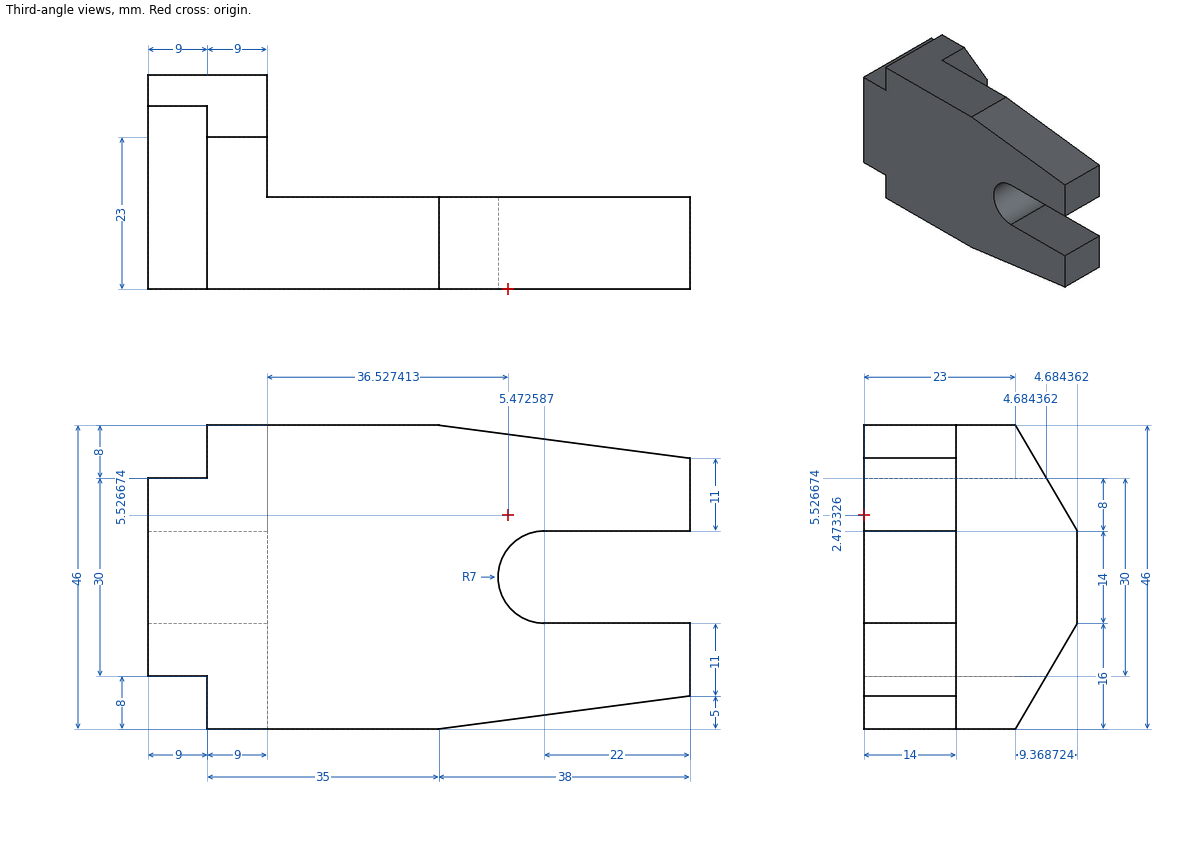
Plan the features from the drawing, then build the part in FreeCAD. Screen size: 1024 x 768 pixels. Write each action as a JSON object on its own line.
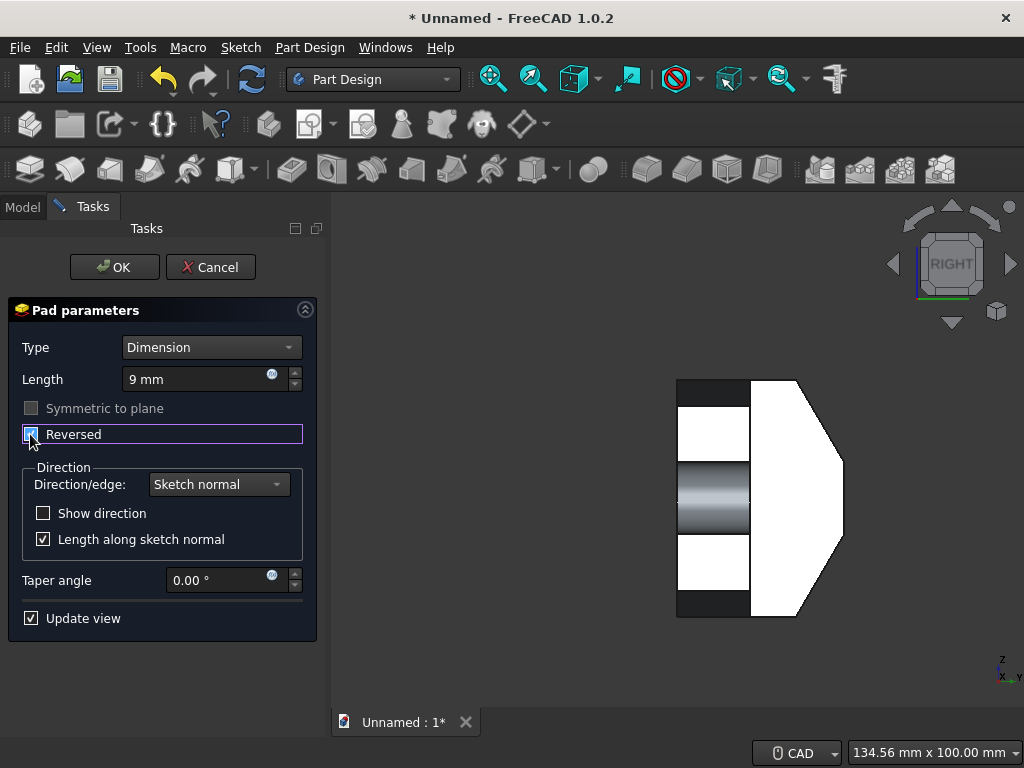
{"action": "left_click", "coordinate": [115, 267]}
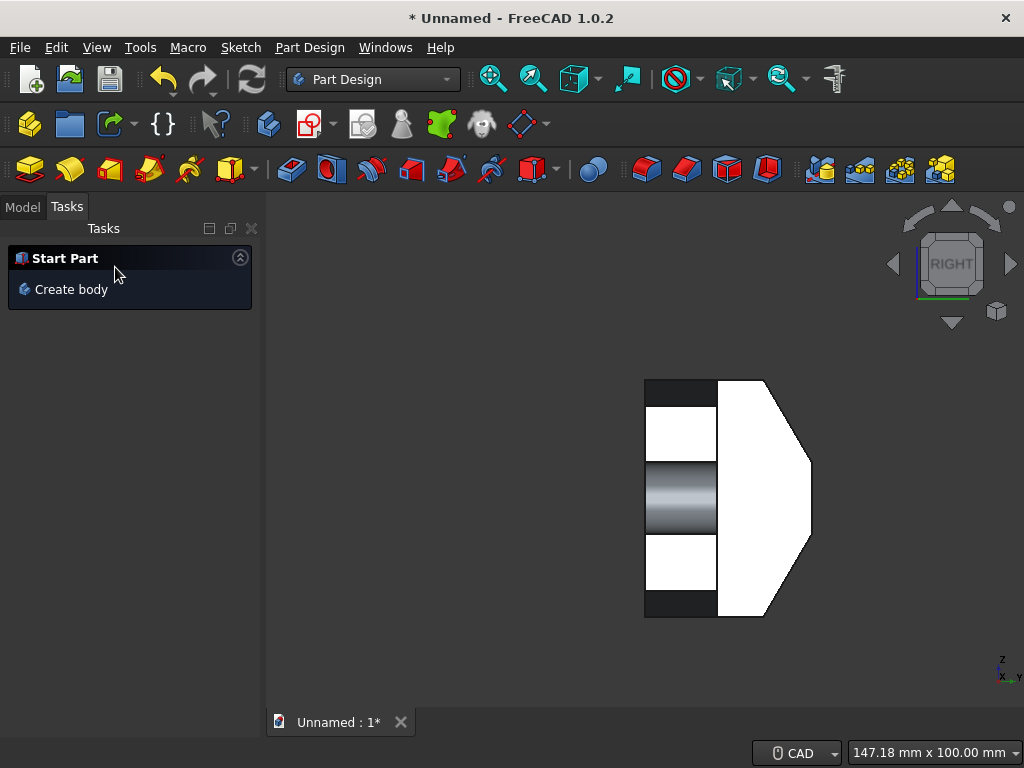
{"action": "key", "text": "6"}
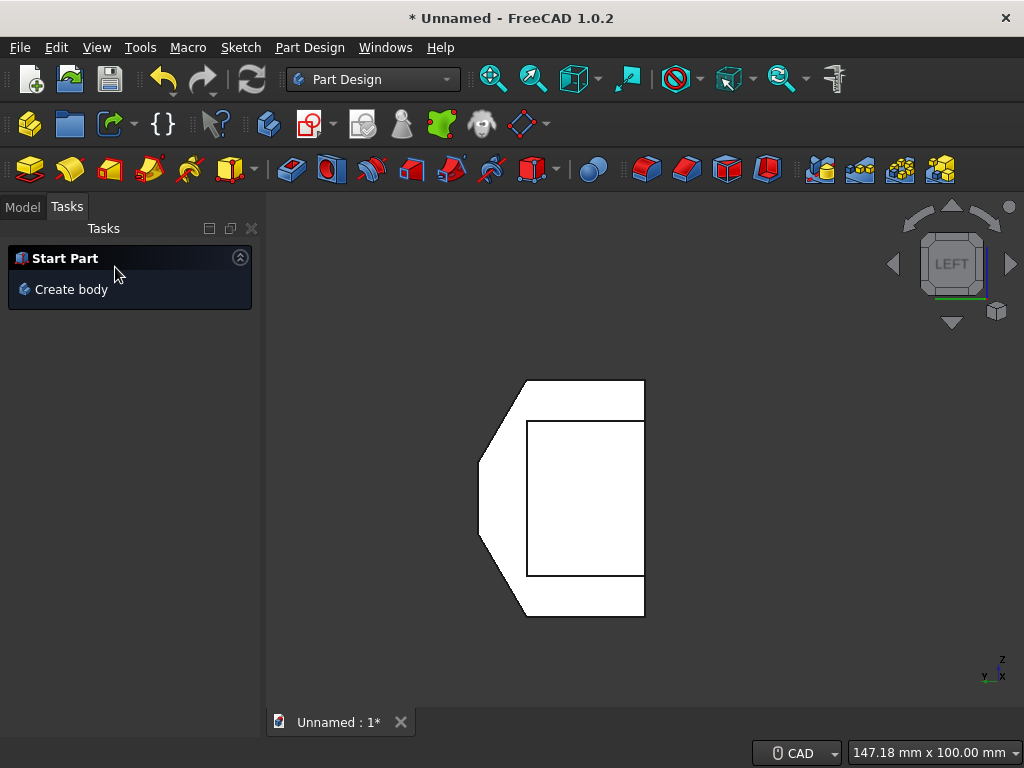
{"action": "left_click", "coordinate": [538, 599]}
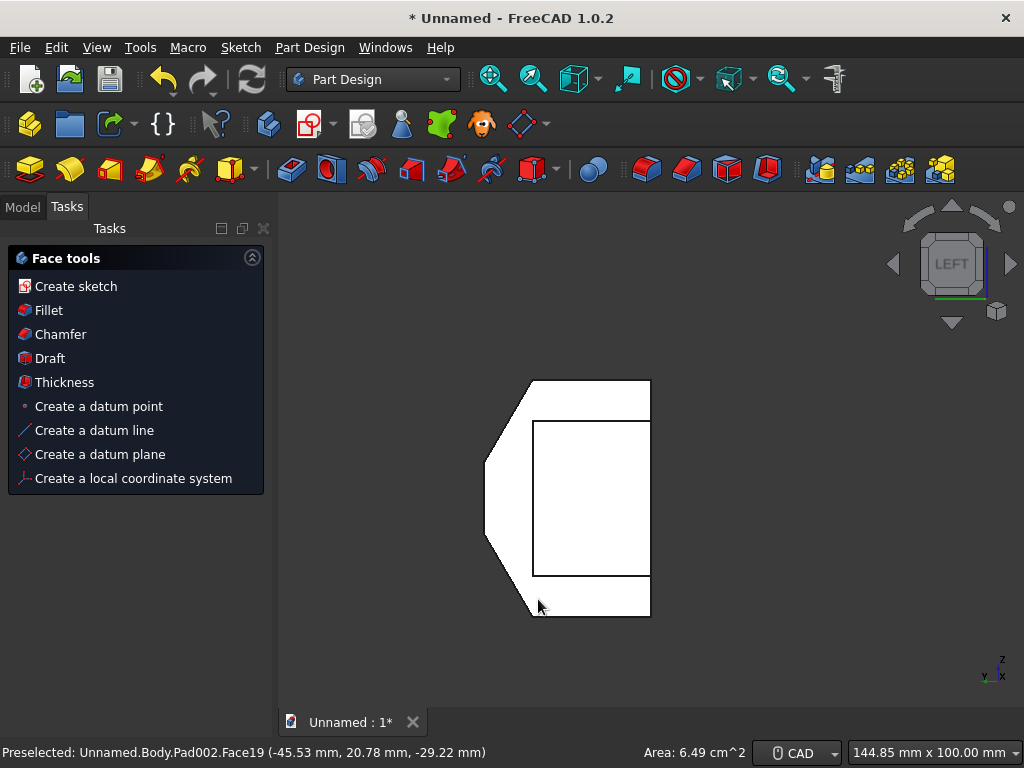
{"action": "left_click", "coordinate": [310, 124]}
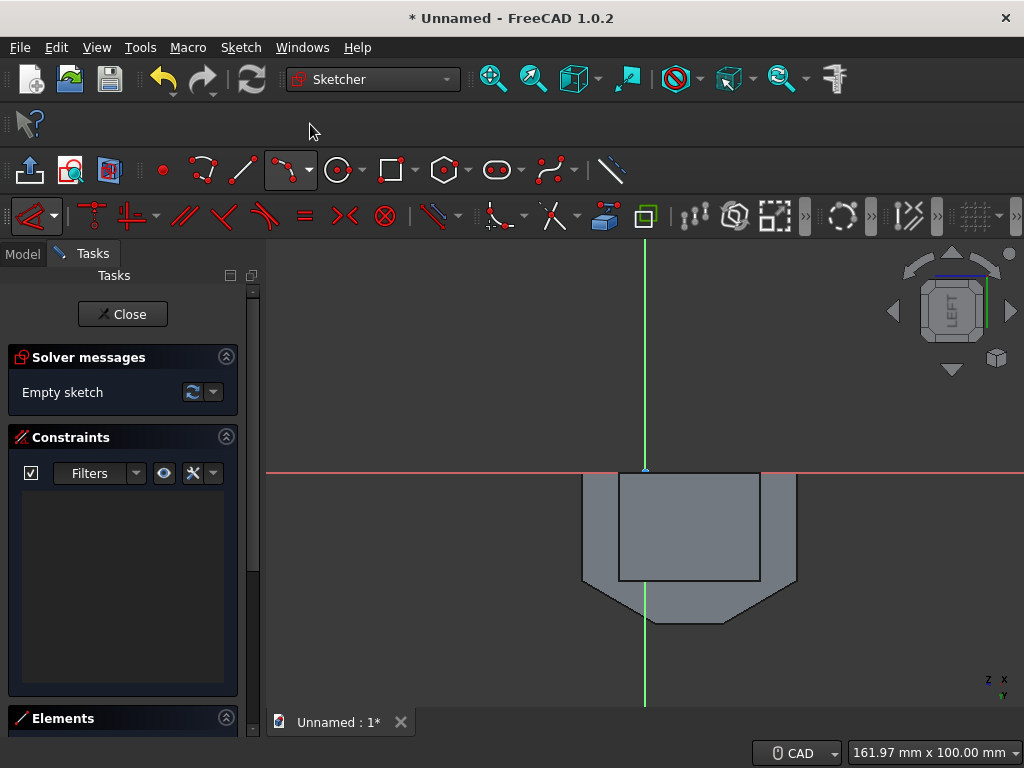
{"action": "scroll", "coordinate": [827, 641], "scroll_direction": "up", "scroll_amount": 3}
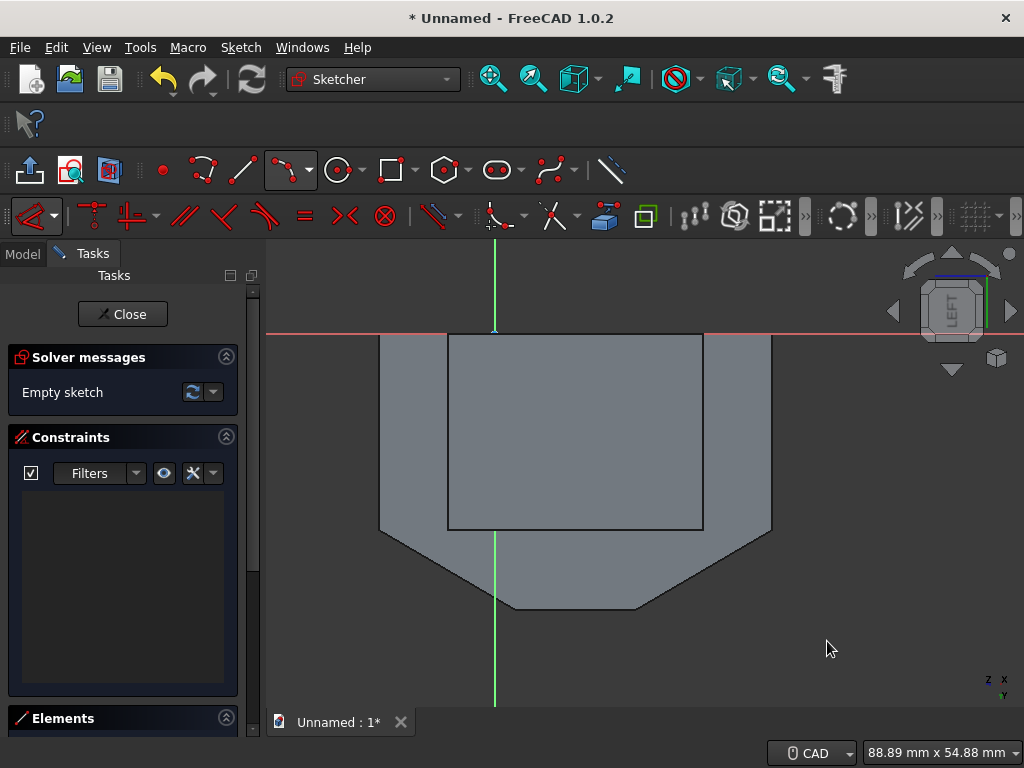
{"action": "left_click", "coordinate": [204, 170]}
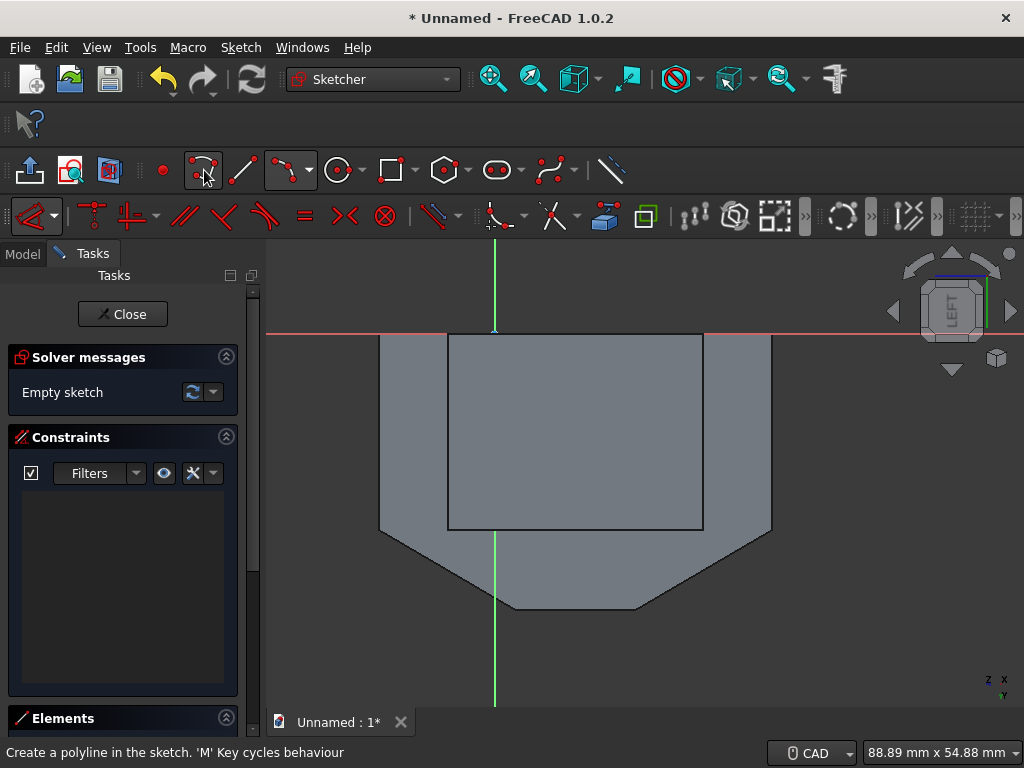
{"action": "left_click", "coordinate": [448, 530]}
{"action": "left_click", "coordinate": [448, 570]}
{"action": "left_click", "coordinate": [516, 610]}
{"action": "left_click", "coordinate": [635, 610]}
{"action": "left_click", "coordinate": [703, 570]}
{"action": "left_click", "coordinate": [703, 530]}
{"action": "left_click", "coordinate": [448, 531]}
{"action": "key", "text": "Escape"}
{"action": "key", "text": "Escape"}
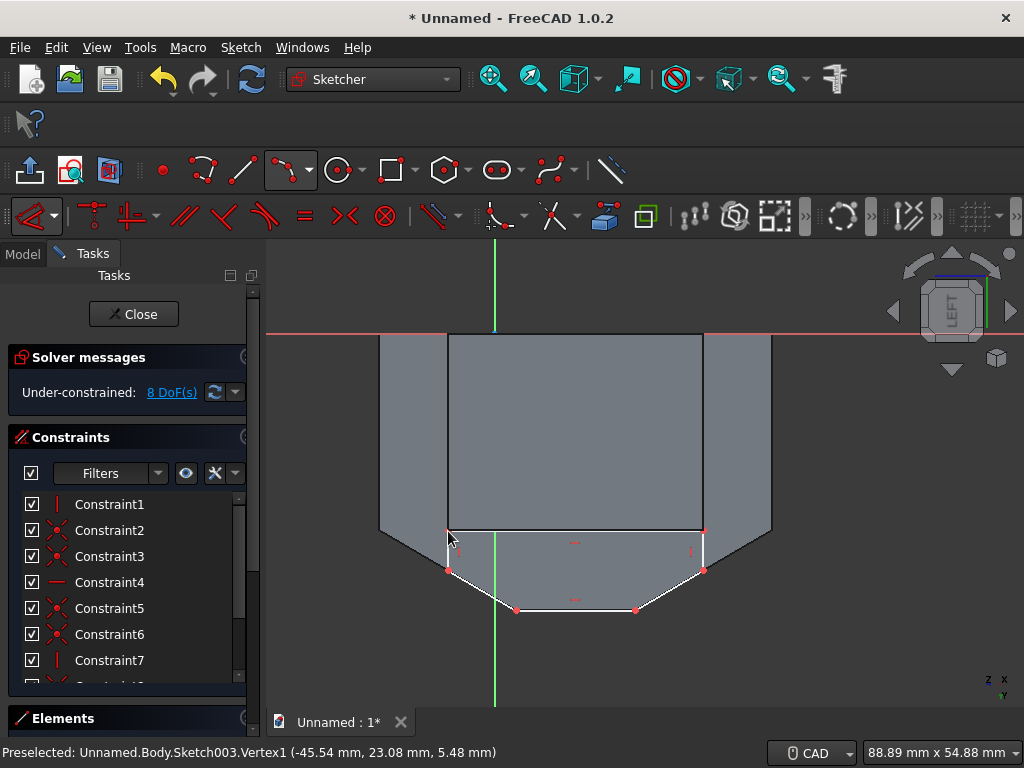
{"action": "left_click", "coordinate": [552, 611]}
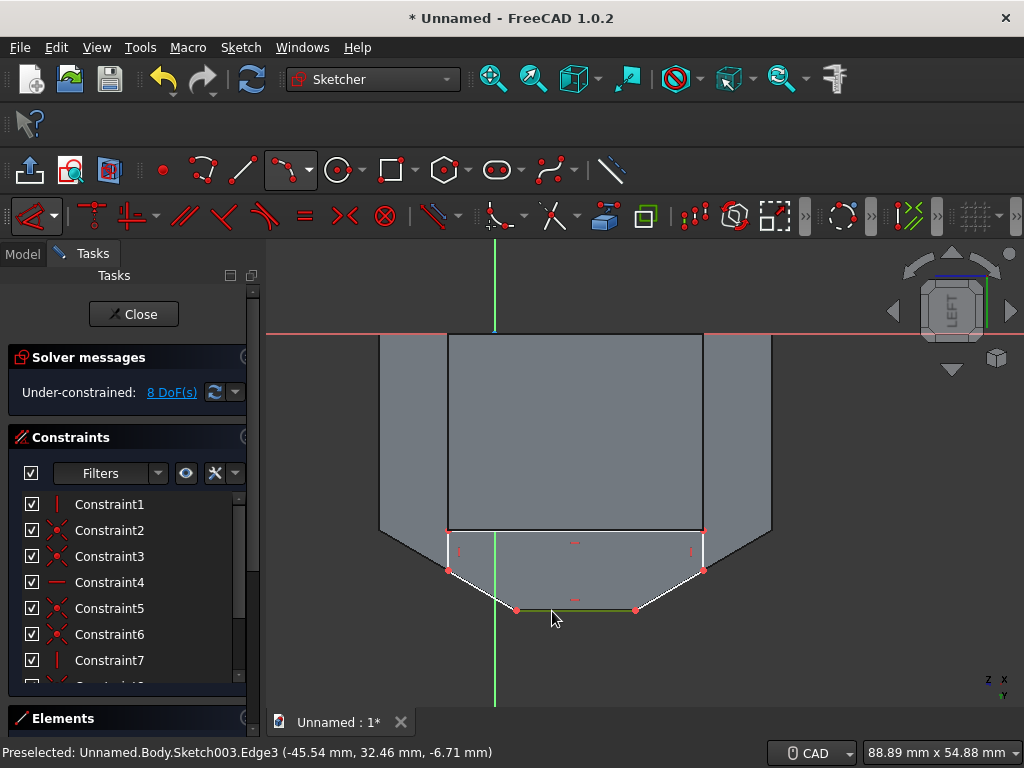
{"action": "left_click", "coordinate": [56, 216]}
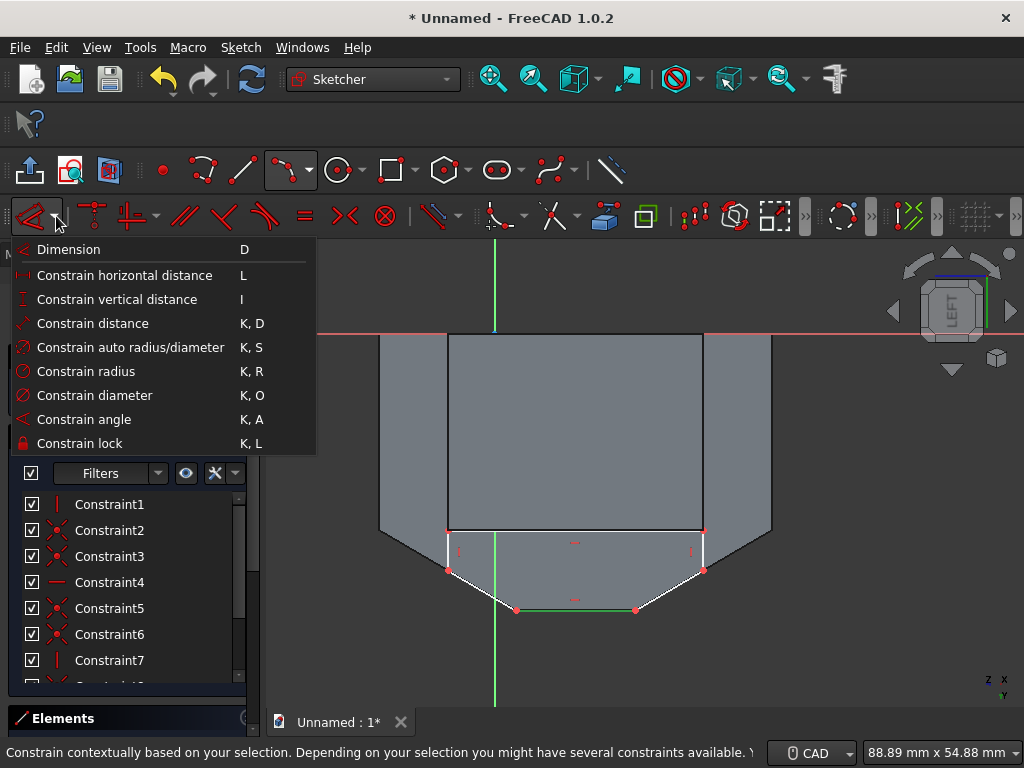
{"action": "left_click", "coordinate": [164, 275]}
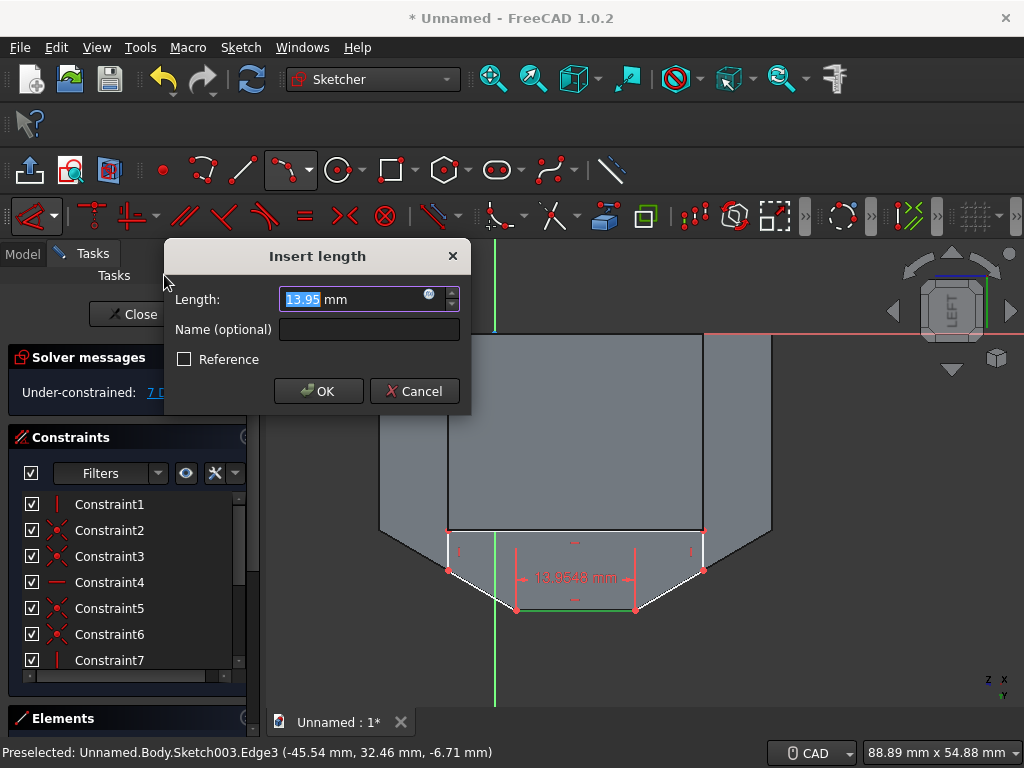
{"action": "type", "text": "14"}
{"action": "key", "text": "Return"}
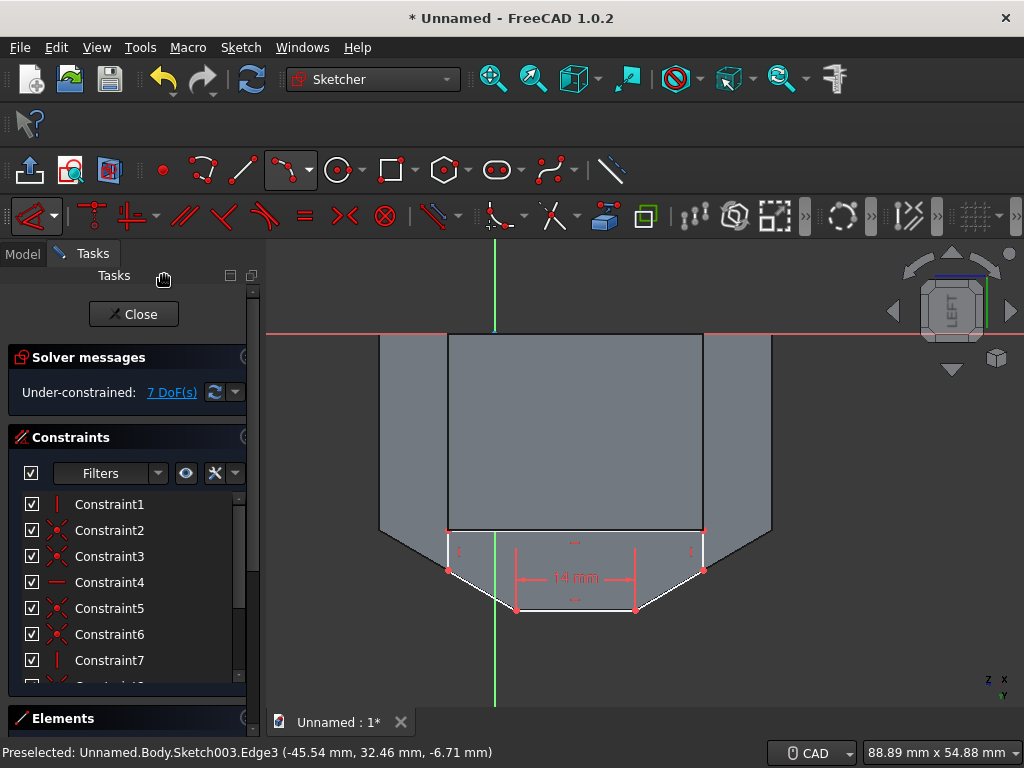
{"action": "left_click", "coordinate": [627, 531]}